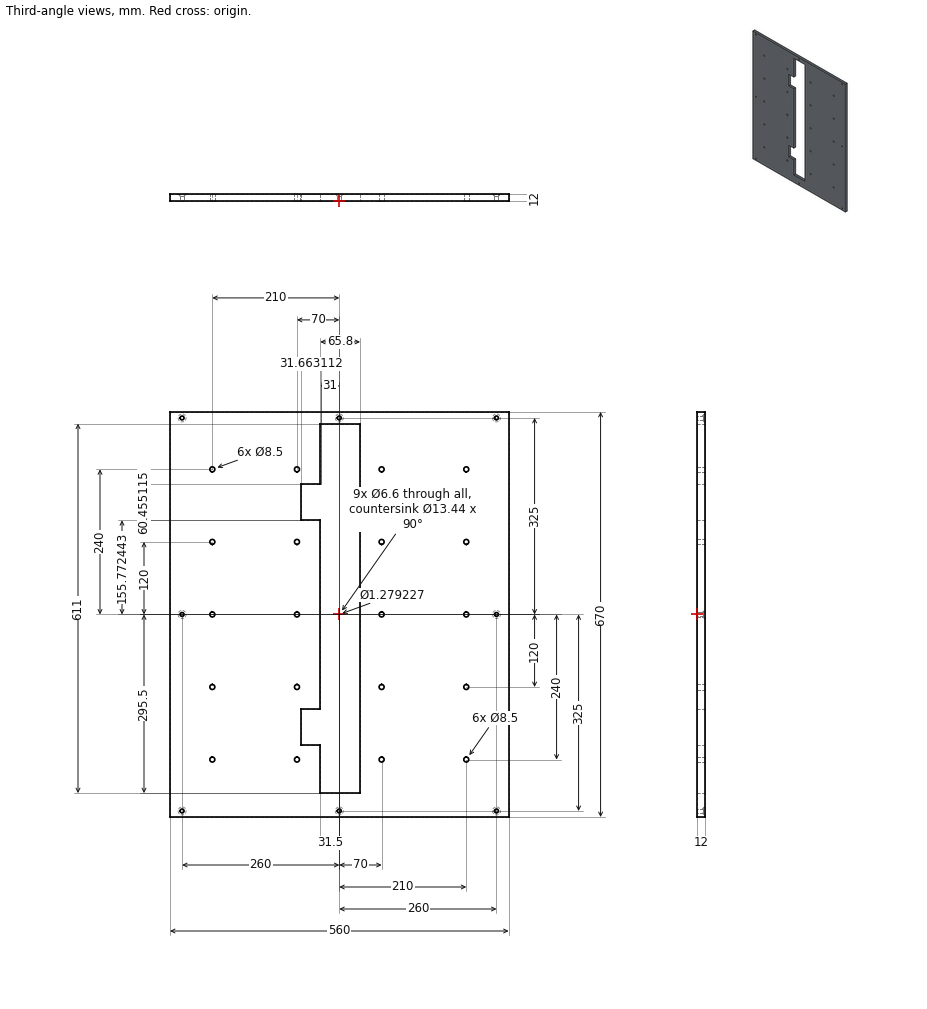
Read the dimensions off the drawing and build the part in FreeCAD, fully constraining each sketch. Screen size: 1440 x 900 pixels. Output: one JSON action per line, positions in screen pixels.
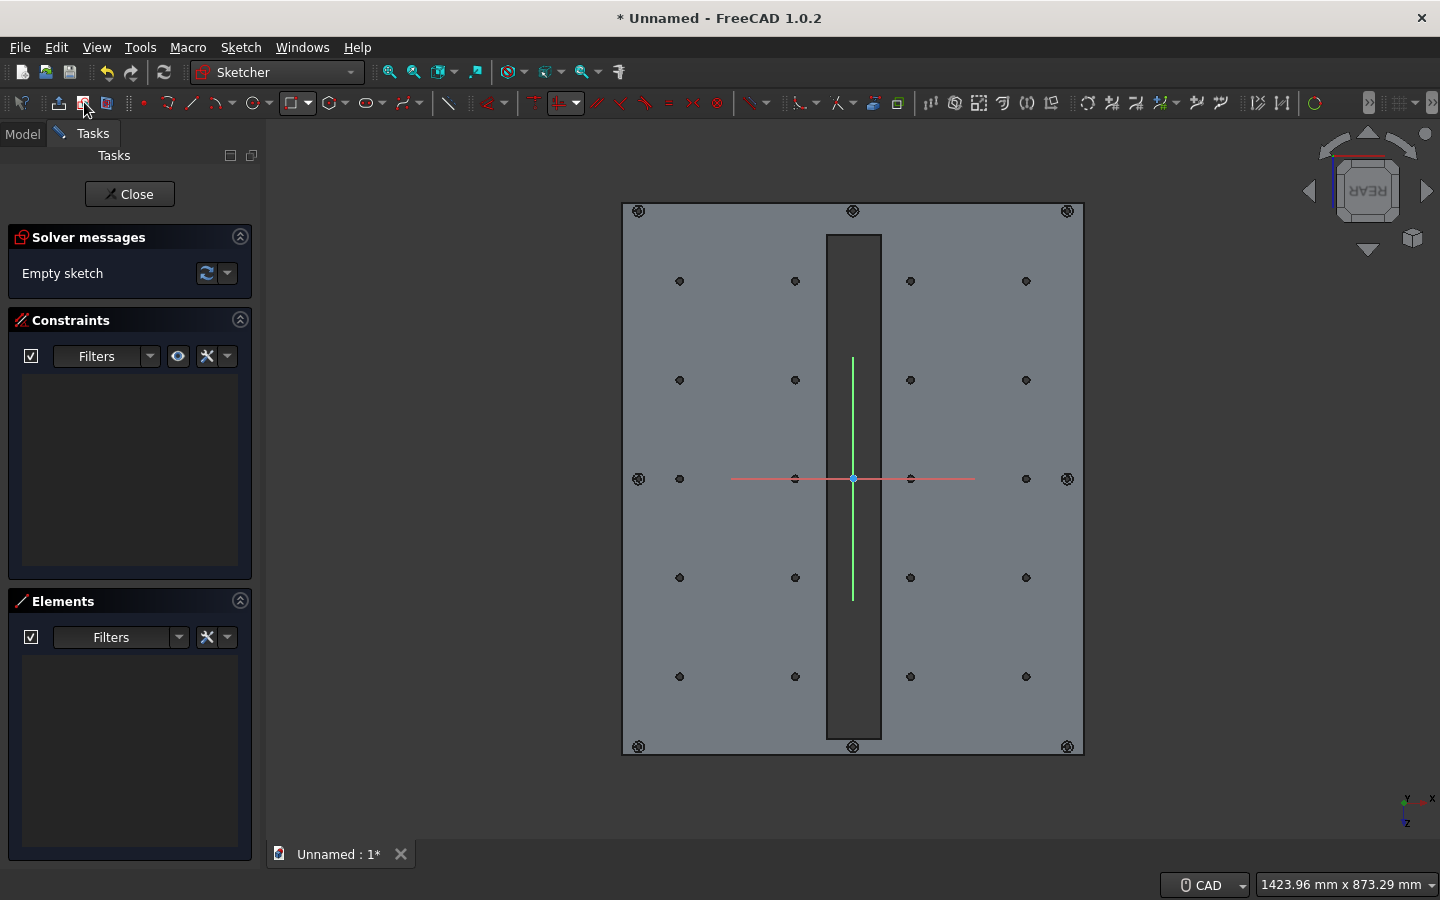
{"action": "scroll", "coordinate": [818, 651], "scroll_direction": "up", "scroll_amount": 11}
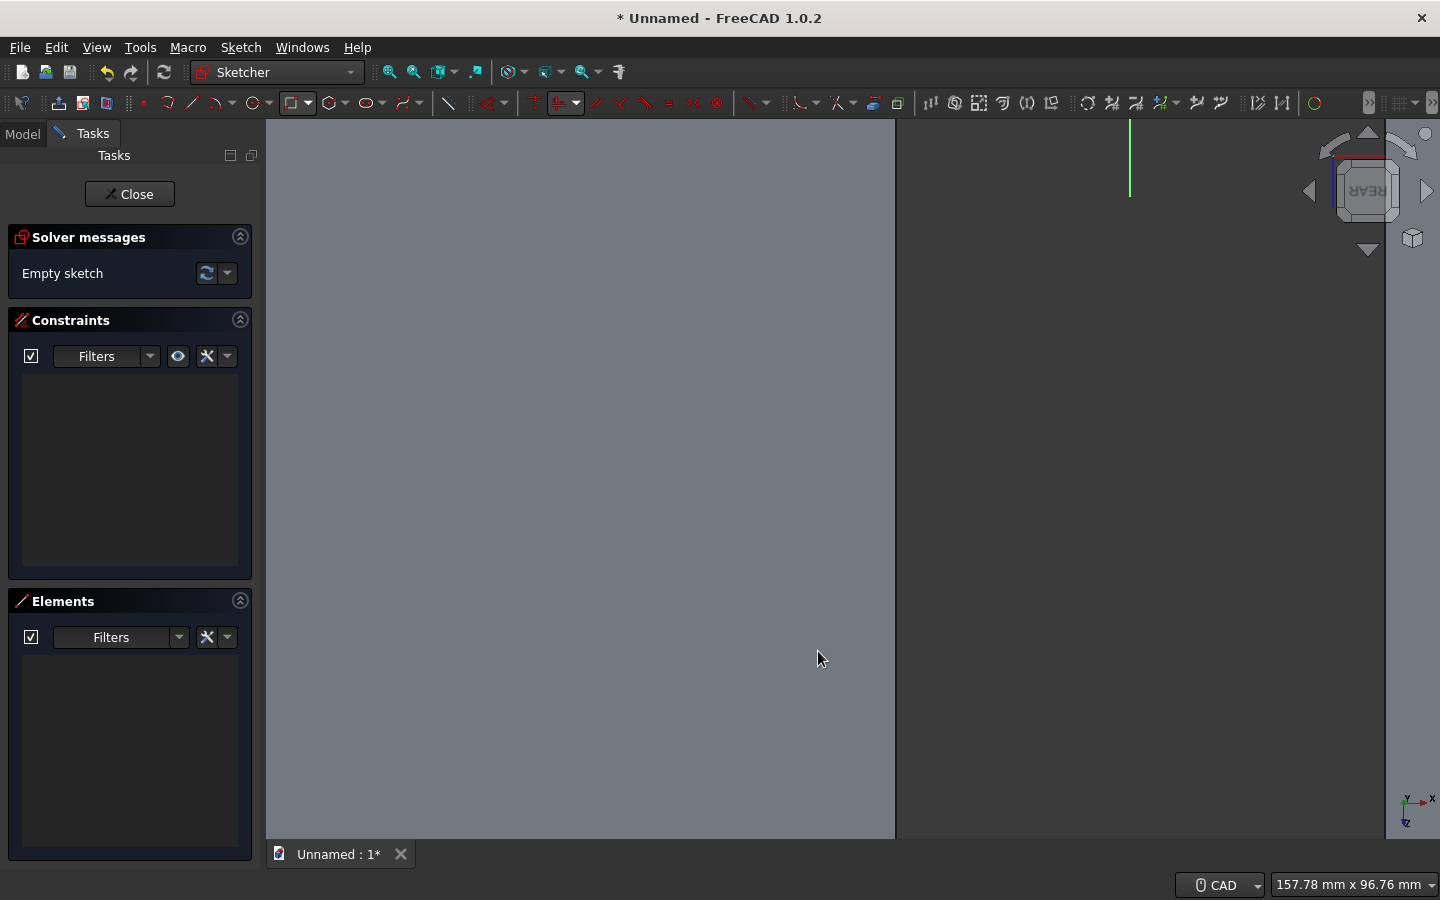
{"action": "left_click", "coordinate": [292, 104]}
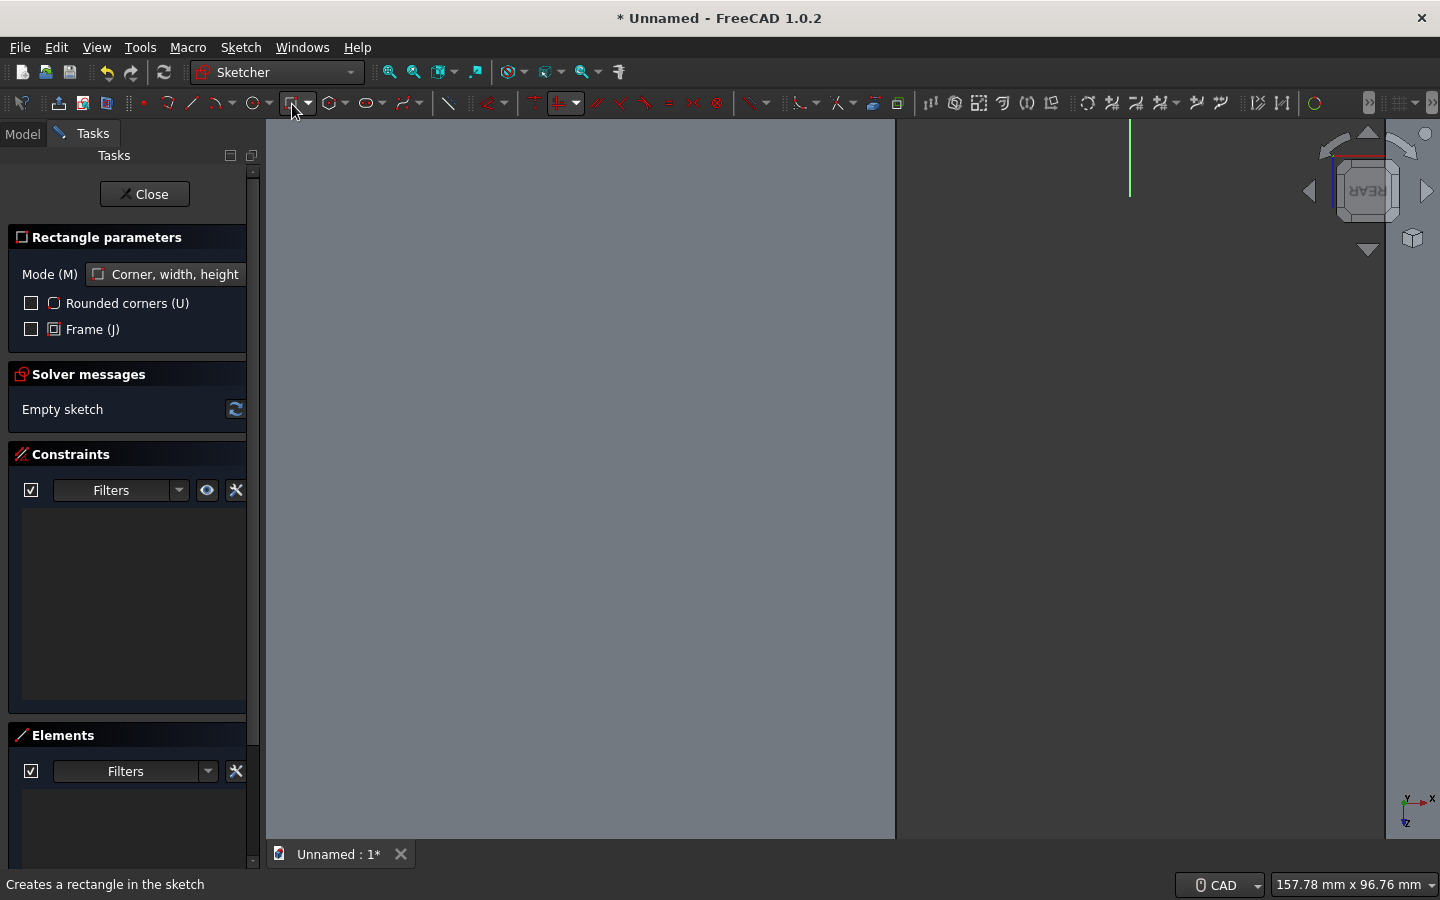
{"action": "left_click", "coordinate": [664, 252]}
{"action": "left_click", "coordinate": [899, 702]}
{"action": "key", "text": "Escape"}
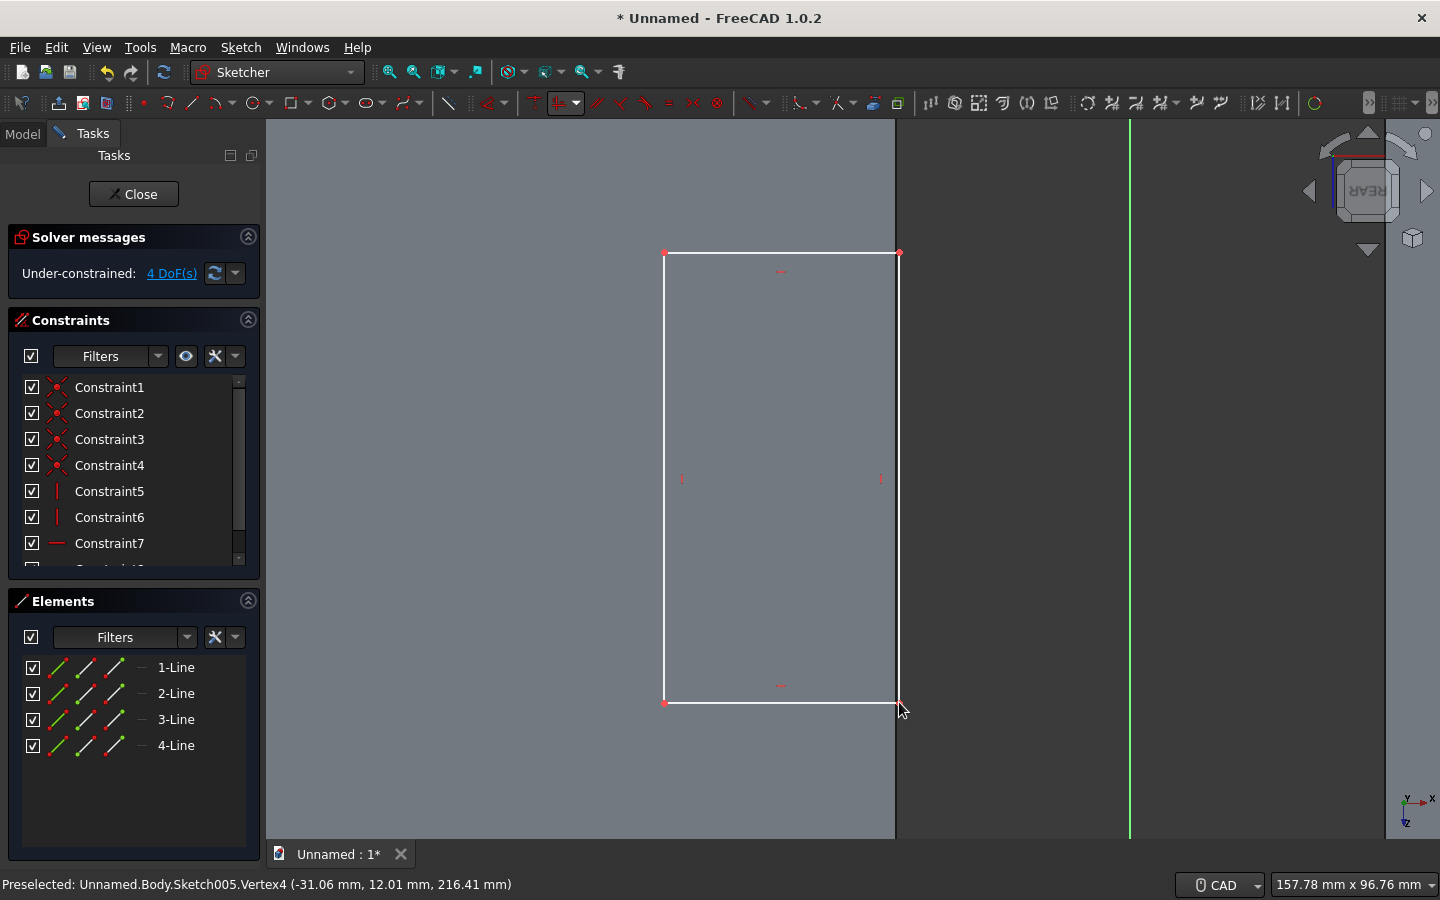
{"action": "left_click", "coordinate": [488, 104]}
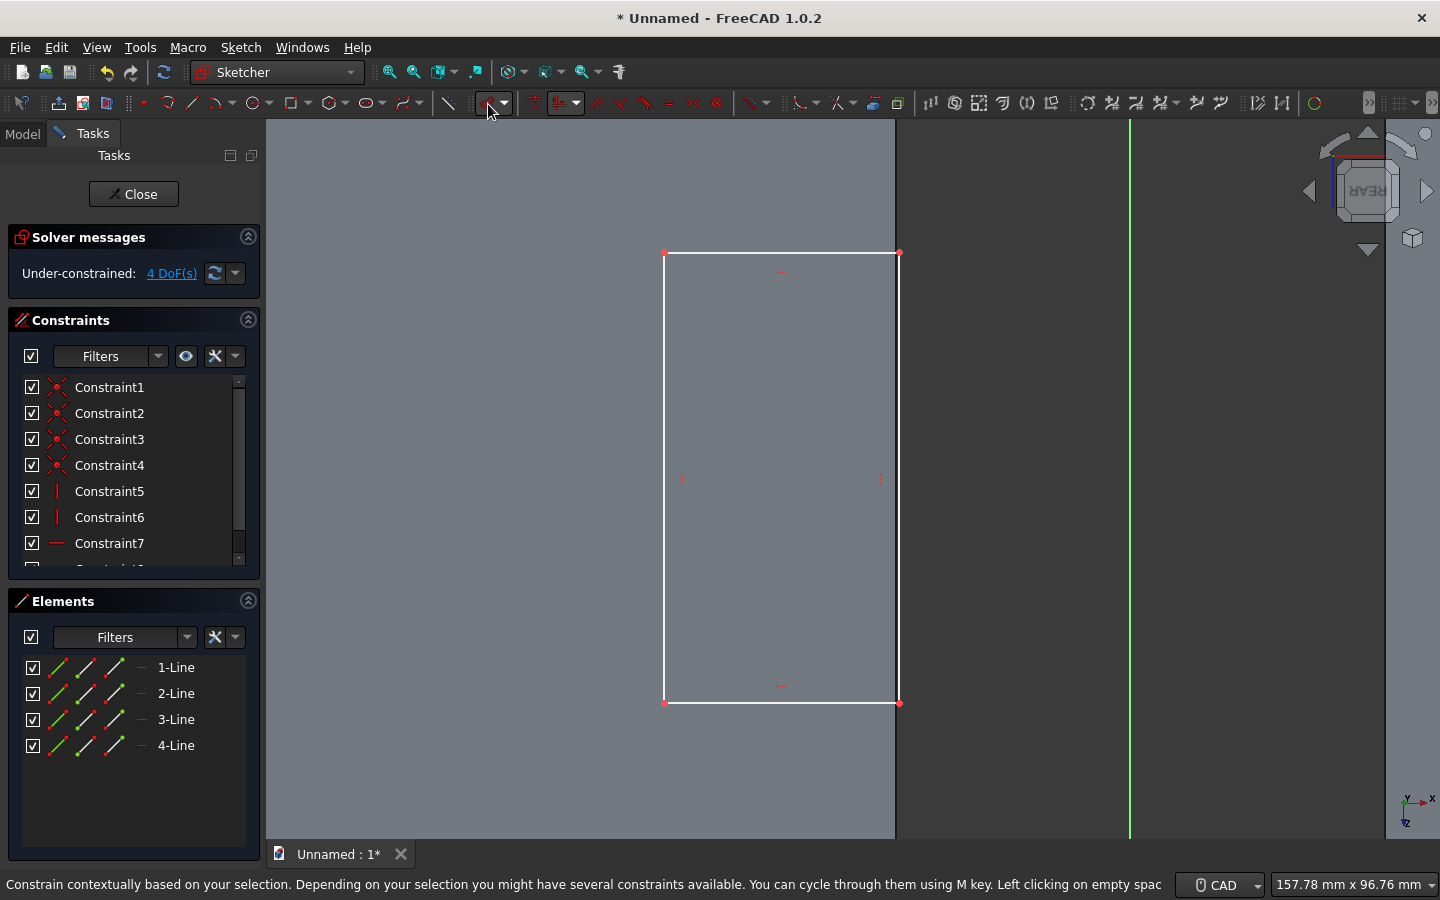
{"action": "left_click", "coordinate": [899, 703]}
{"action": "left_click", "coordinate": [1015, 737]}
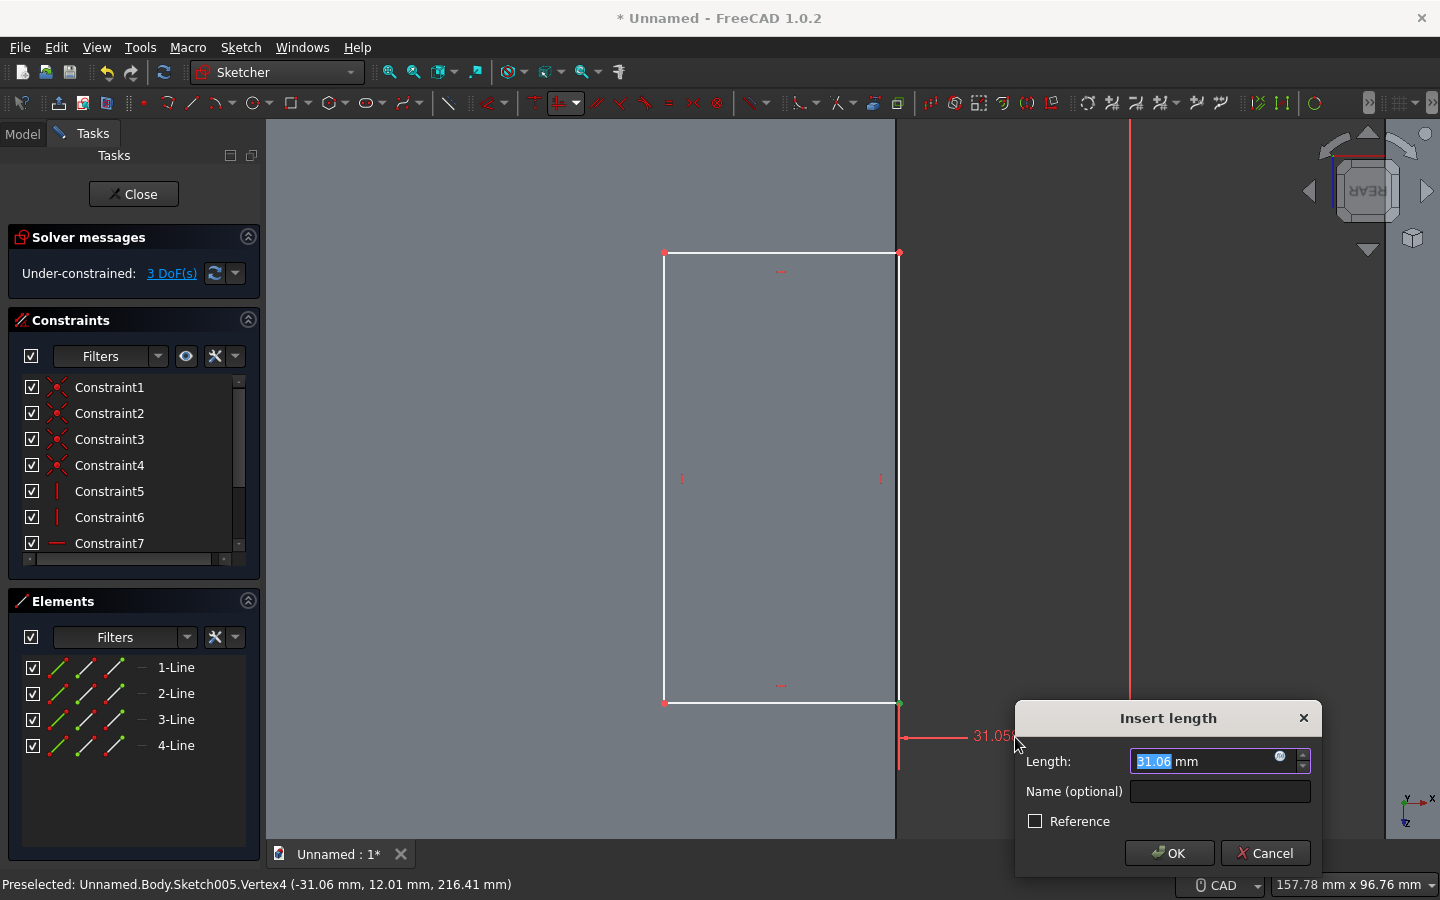
{"action": "type", "text": "31"}
{"action": "key", "text": "Return"}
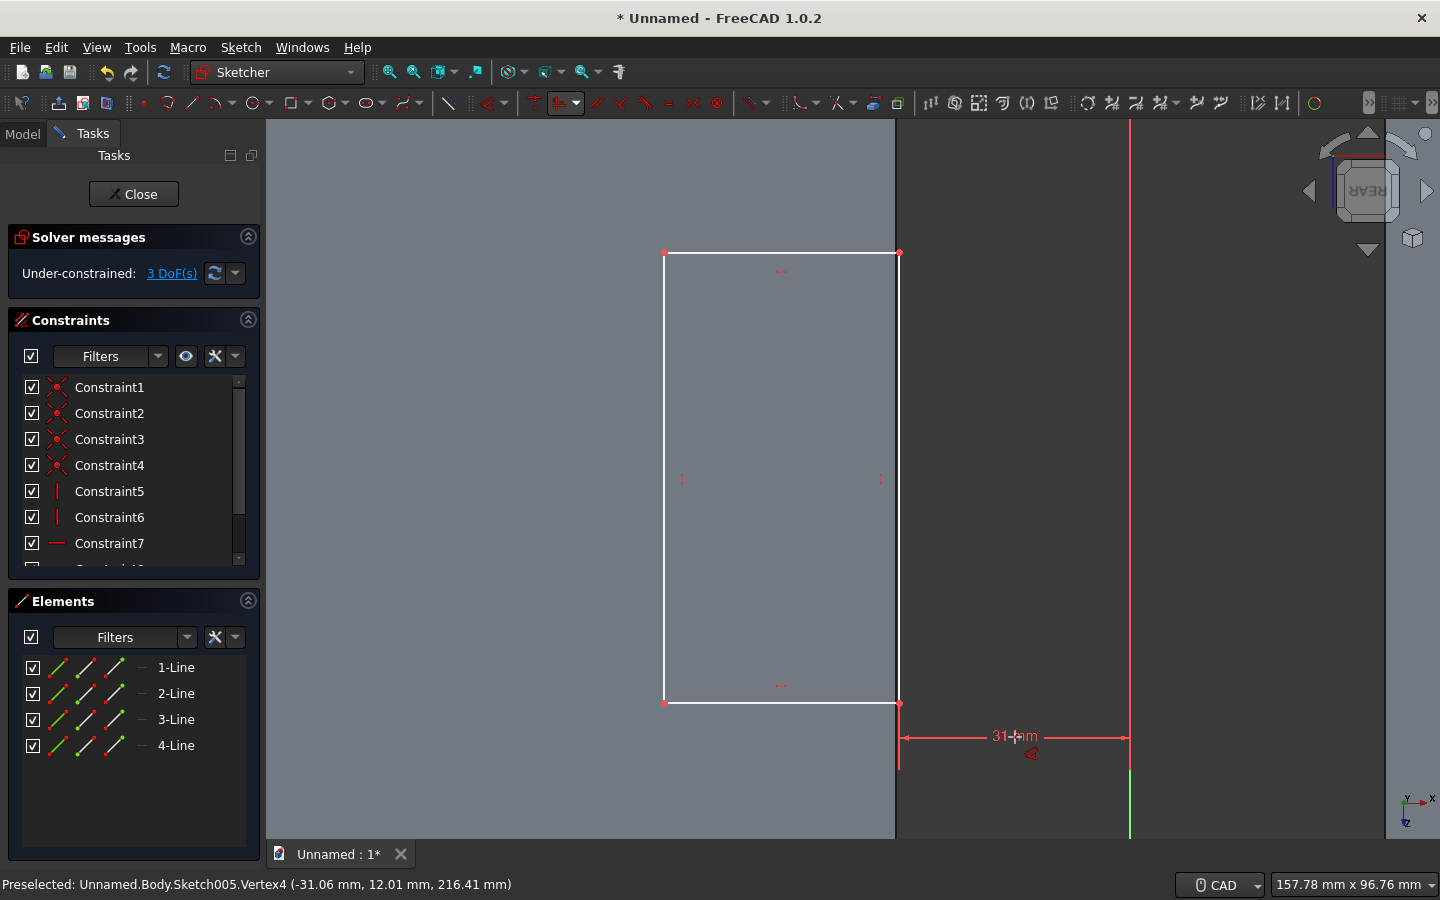
{"action": "left_click", "coordinate": [664, 388]}
{"action": "left_click", "coordinate": [630, 478]}